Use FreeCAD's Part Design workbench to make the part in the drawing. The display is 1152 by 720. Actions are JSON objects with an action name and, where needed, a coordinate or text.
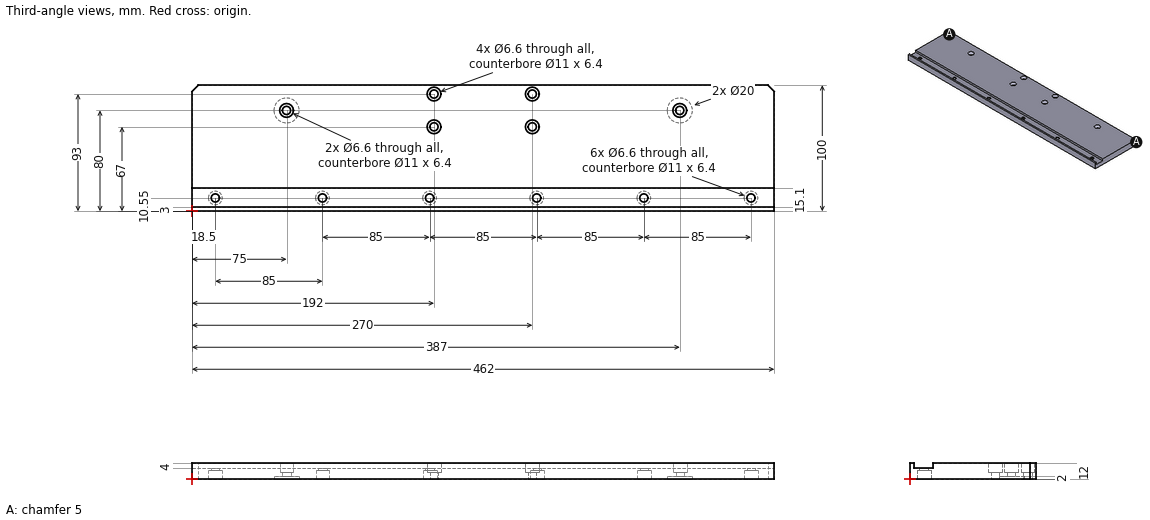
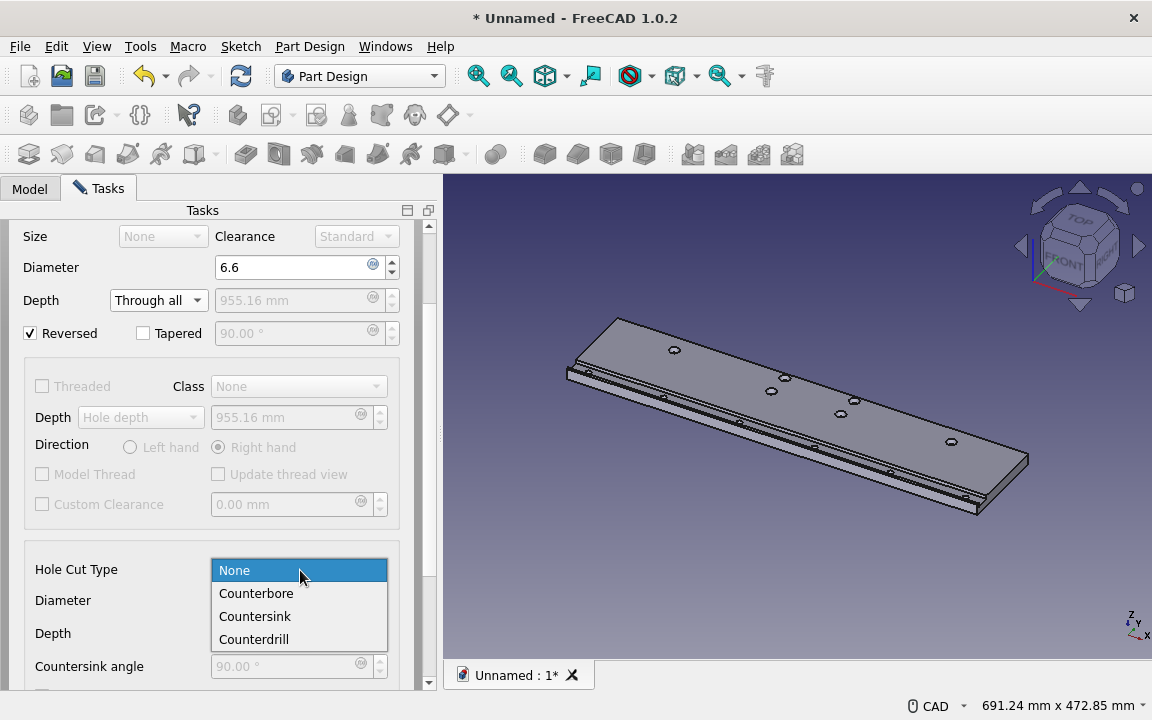
{"action": "left_click", "coordinate": [298, 594]}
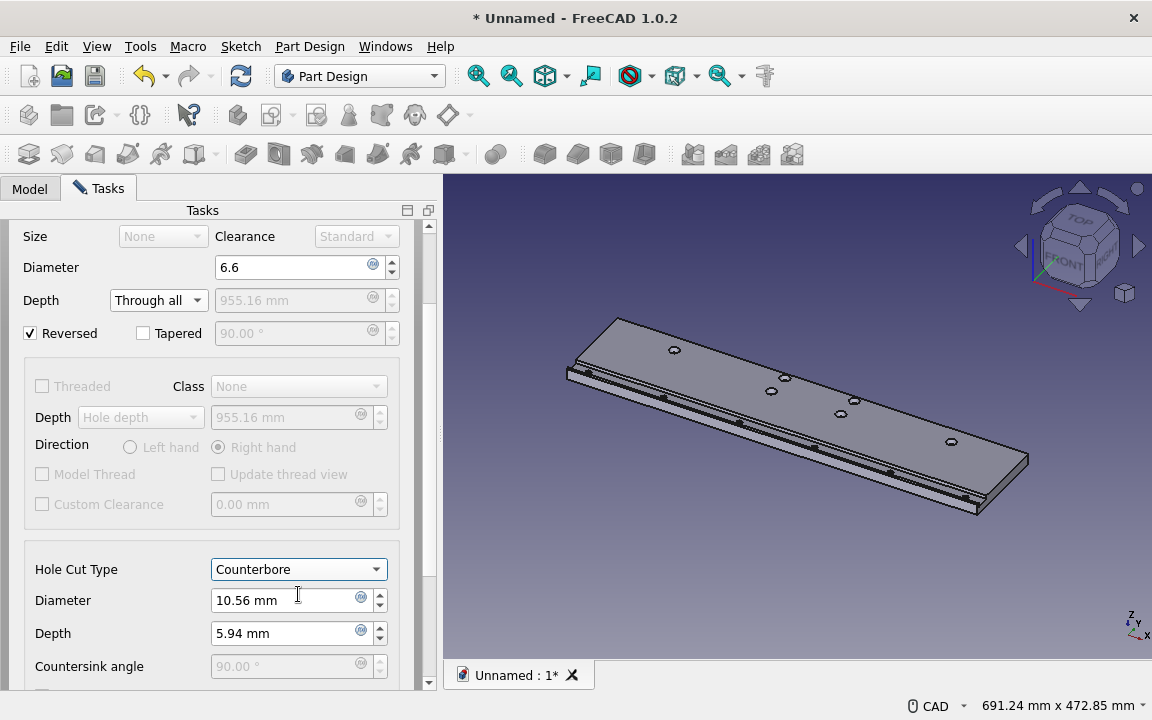
{"action": "triple_click", "coordinate": [292, 600]}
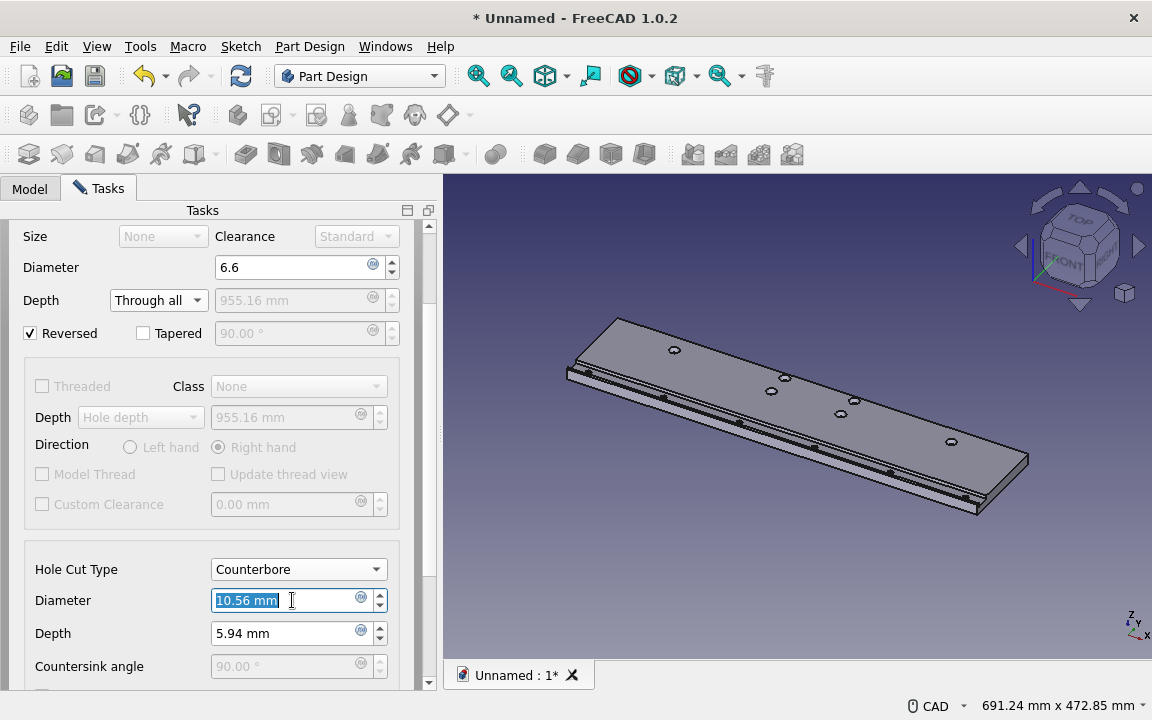
{"action": "type", "text": "11"}
{"action": "key", "text": "Tab"}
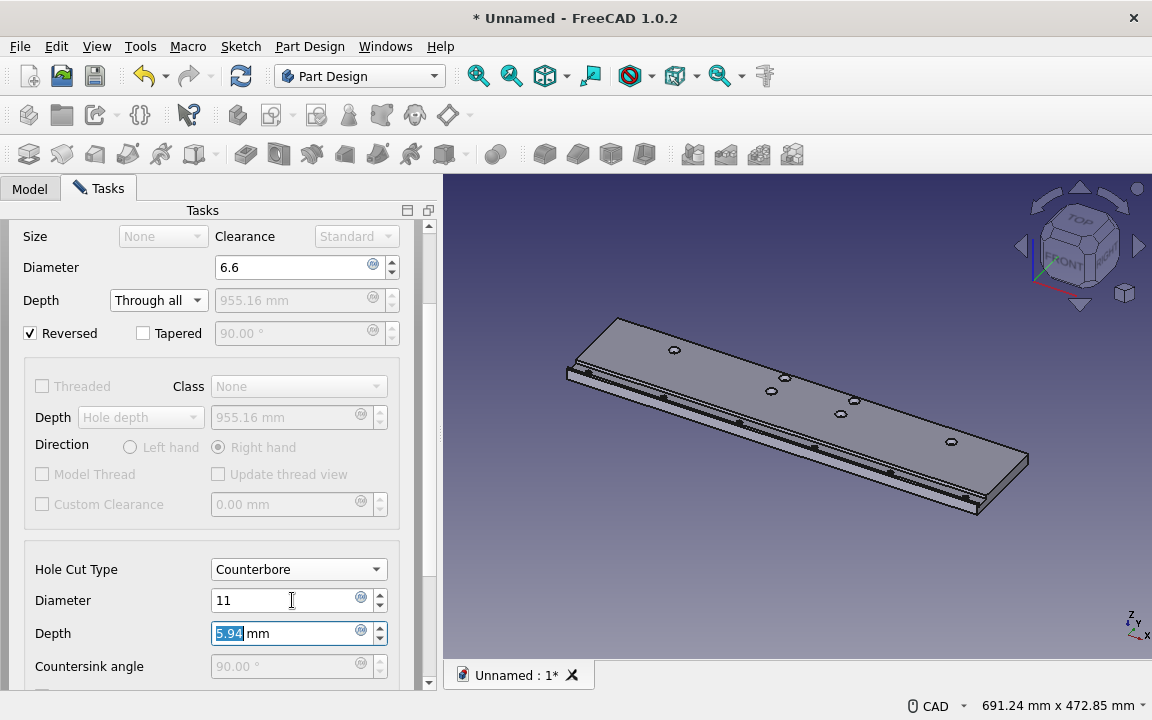
{"action": "type", "text": "6.4"}
{"action": "key", "text": "Tab"}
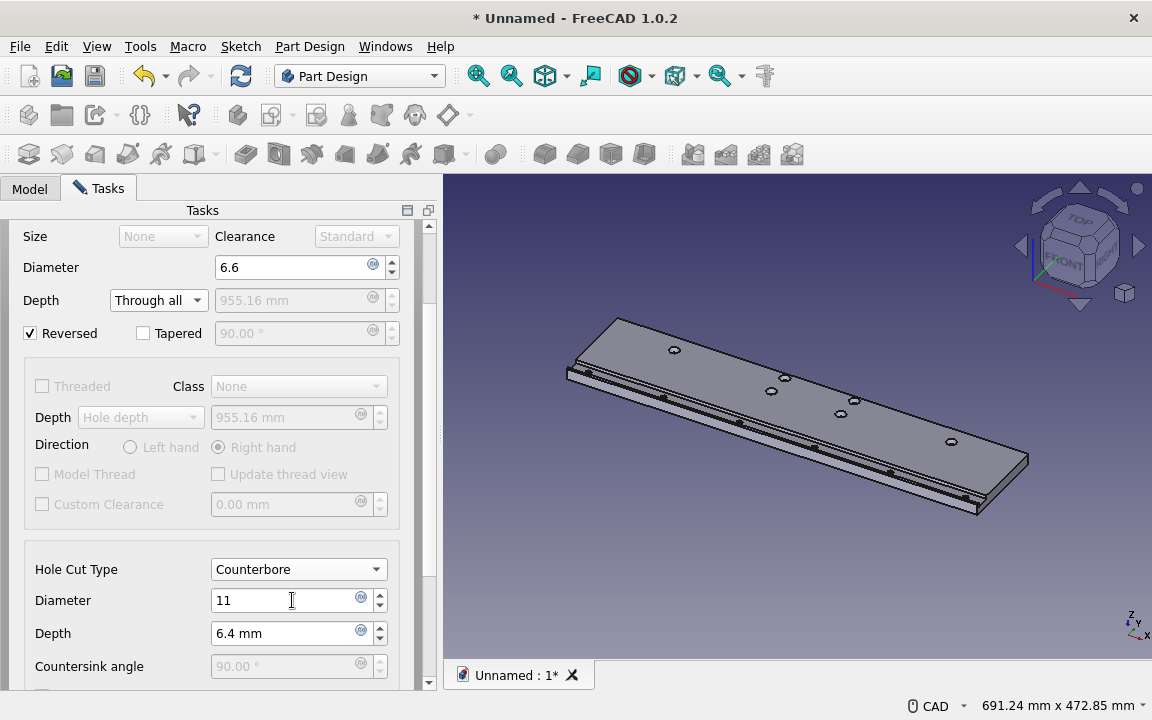
{"action": "scroll", "coordinate": [429, 455], "scroll_direction": "up", "scroll_amount": 3}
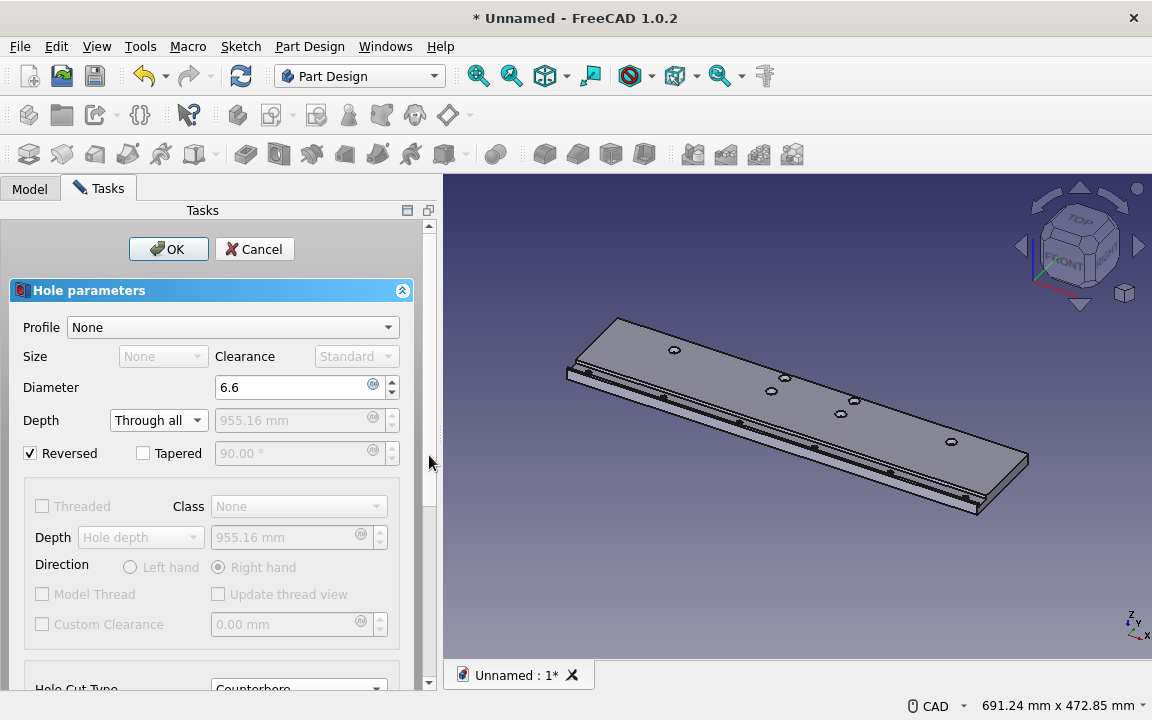
{"action": "left_click", "coordinate": [169, 249]}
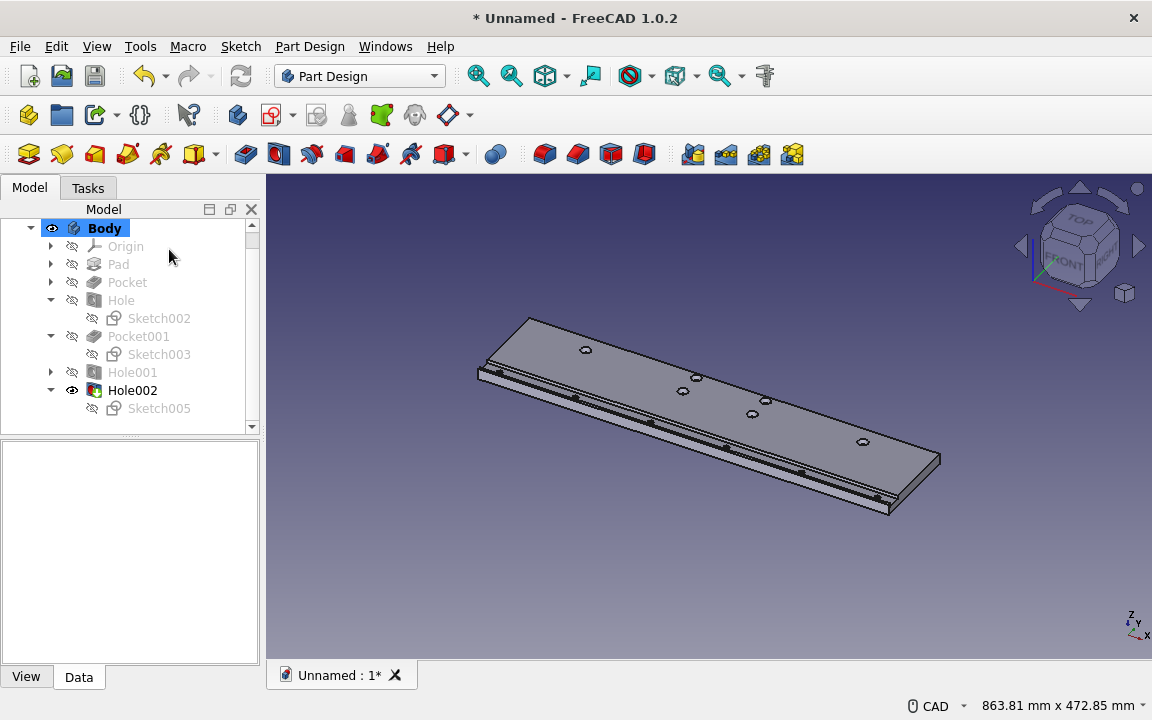
{"action": "scroll", "coordinate": [529, 322], "scroll_direction": "up", "scroll_amount": 6}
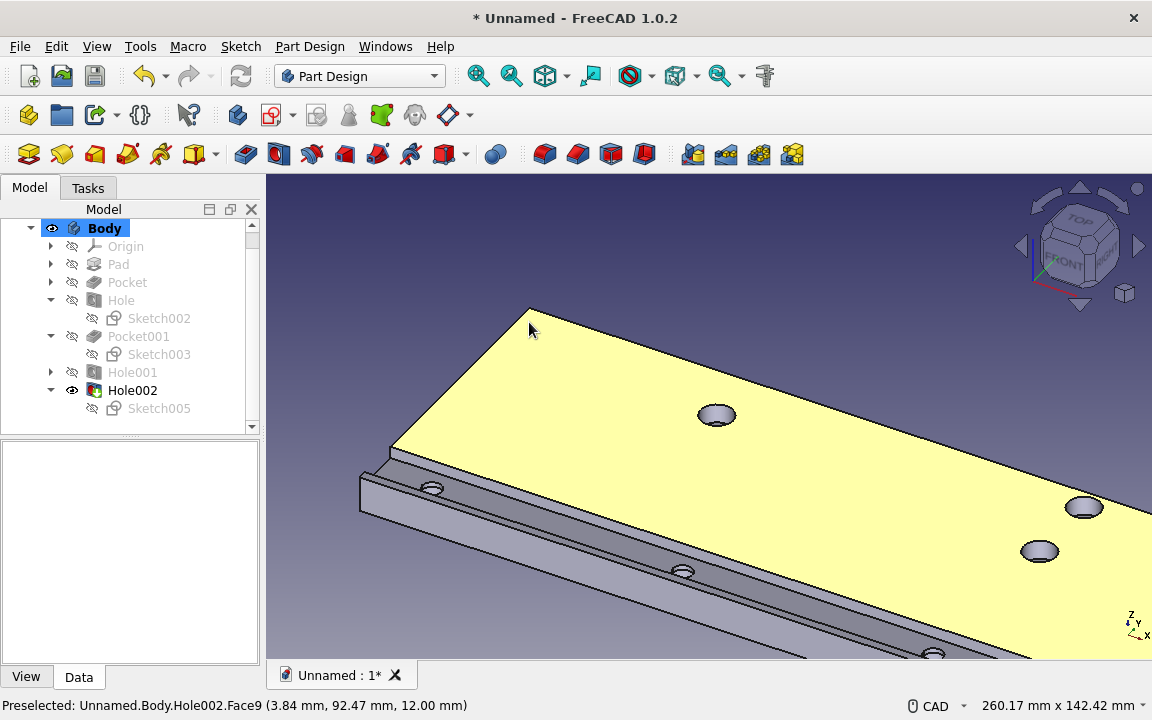
{"action": "left_click", "coordinate": [479, 76]}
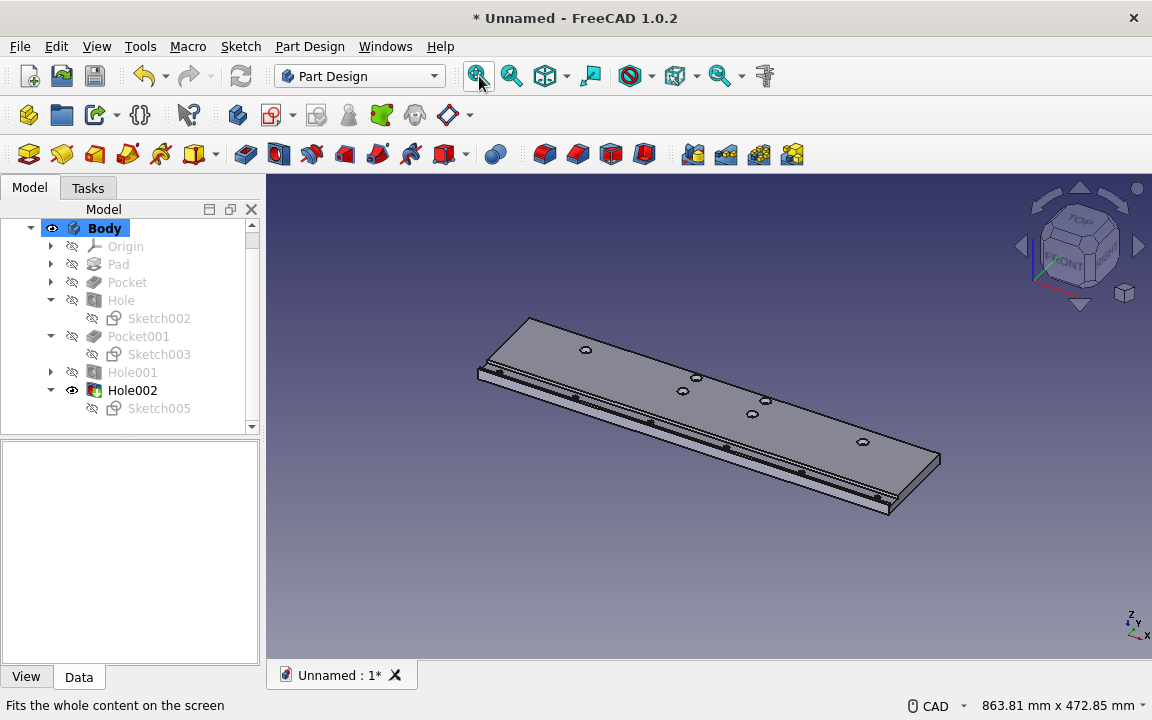
{"action": "key", "text": "0"}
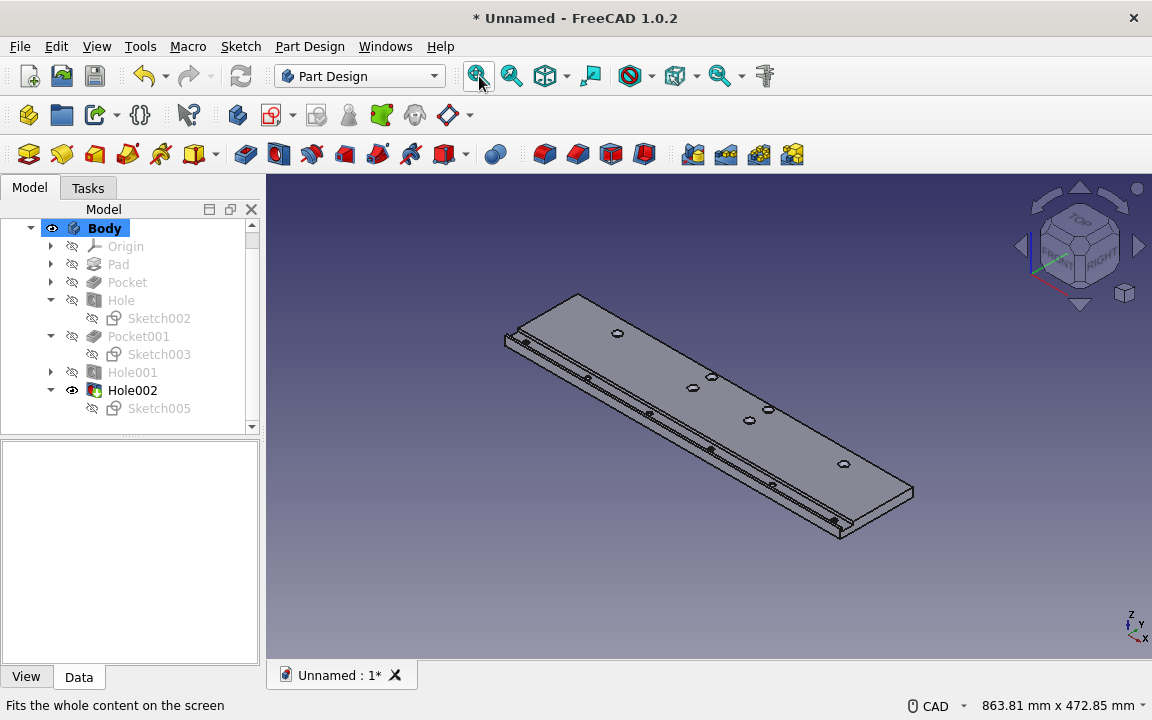
{"action": "scroll", "coordinate": [578, 298], "scroll_direction": "up", "scroll_amount": 6}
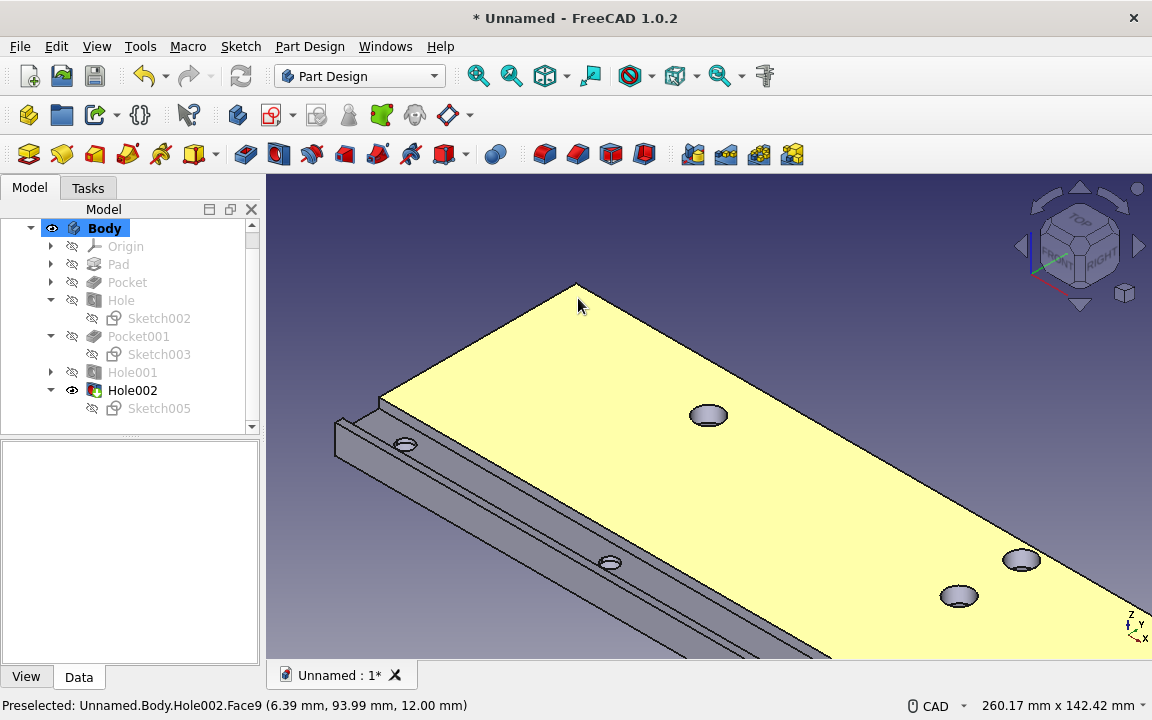
{"action": "left_click", "coordinate": [479, 76]}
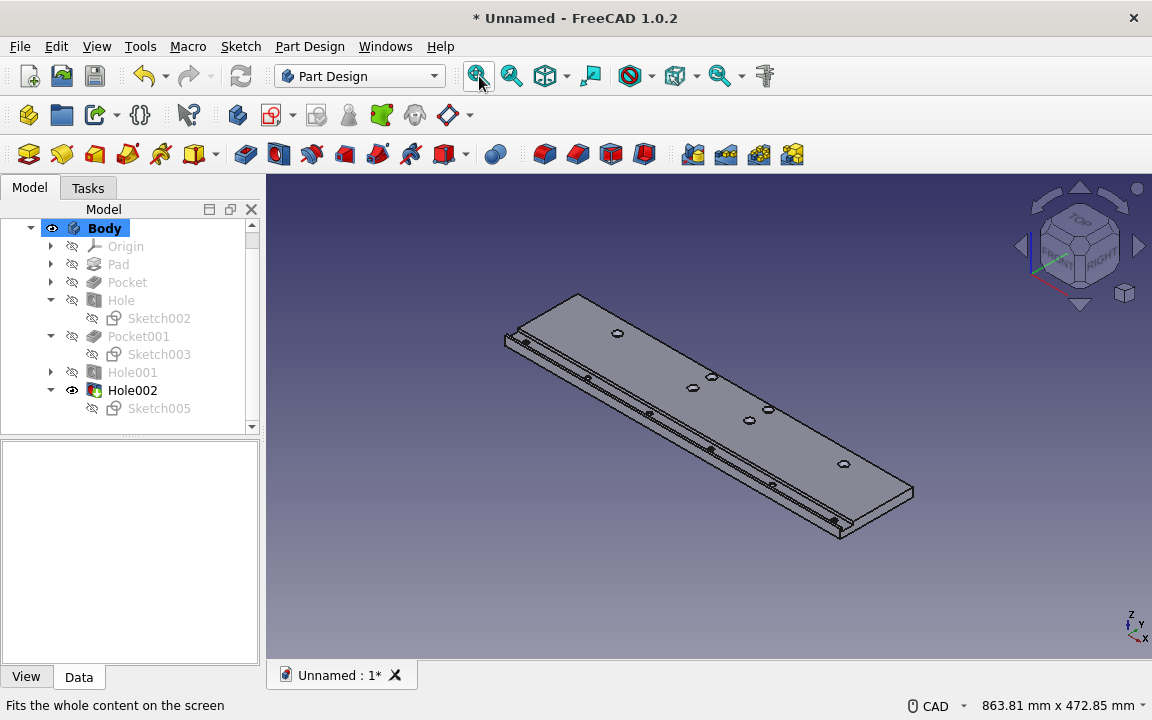
{"action": "key", "text": "2"}